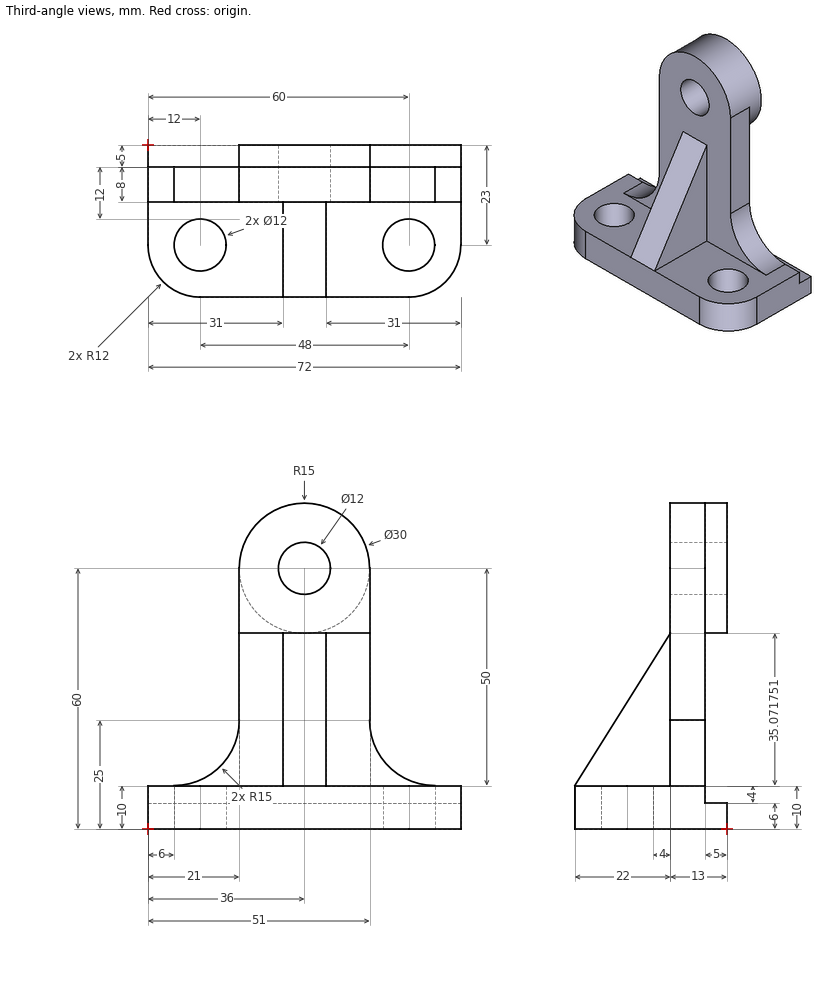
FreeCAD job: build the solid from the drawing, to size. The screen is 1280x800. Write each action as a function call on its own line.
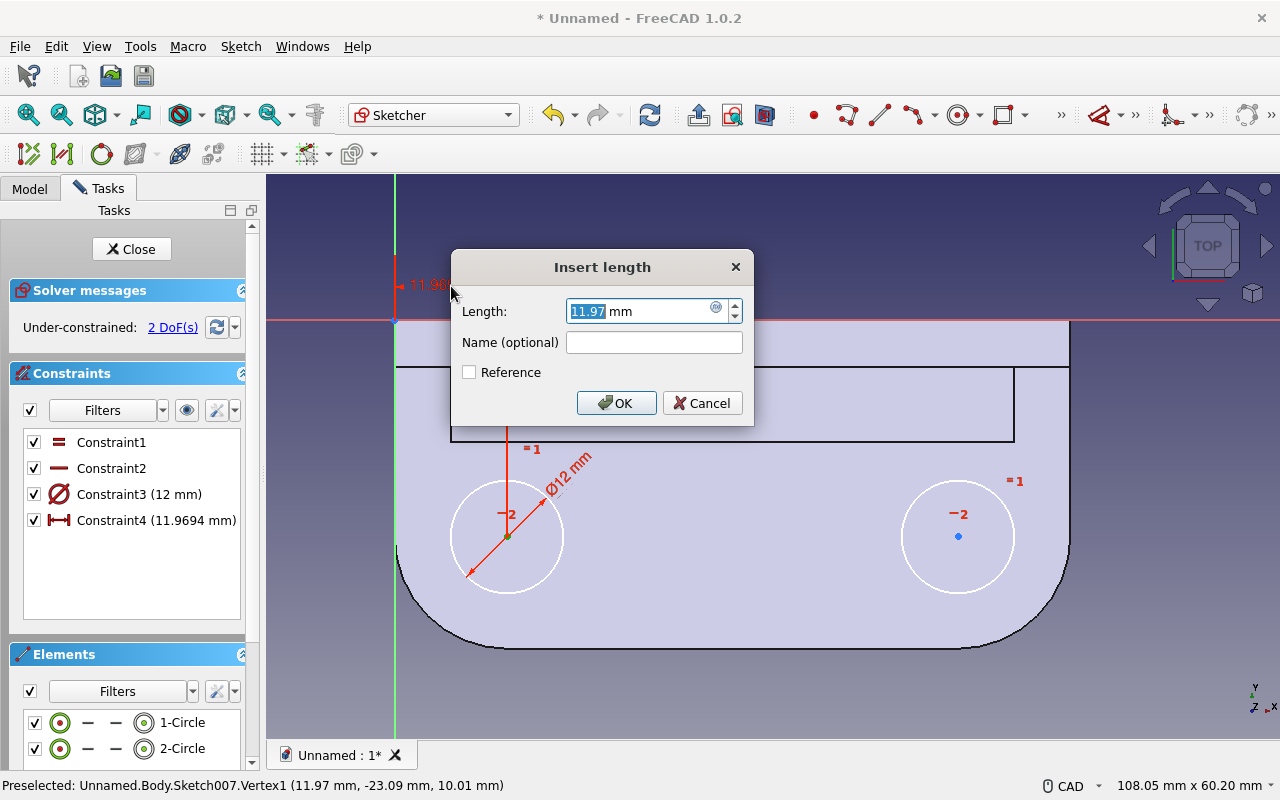
text(12)
key(Return)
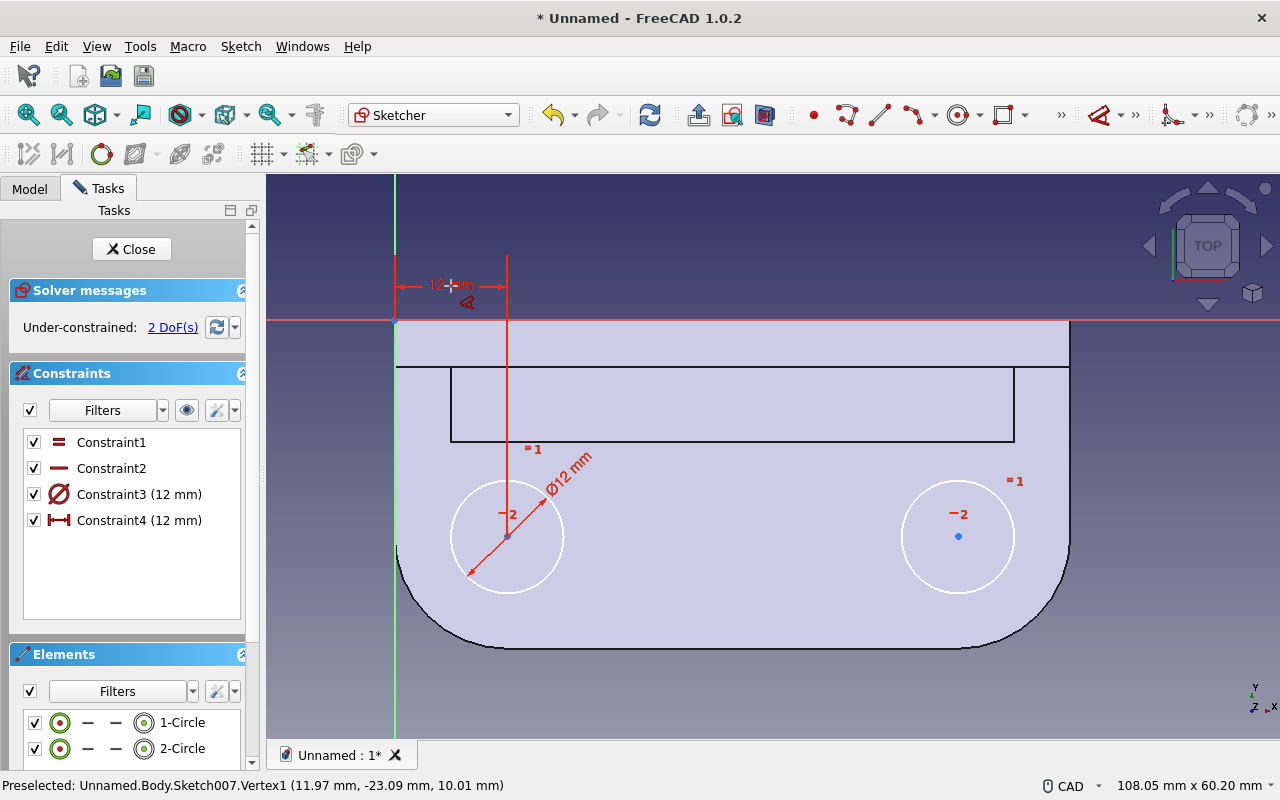
click(507, 537)
click(361, 429)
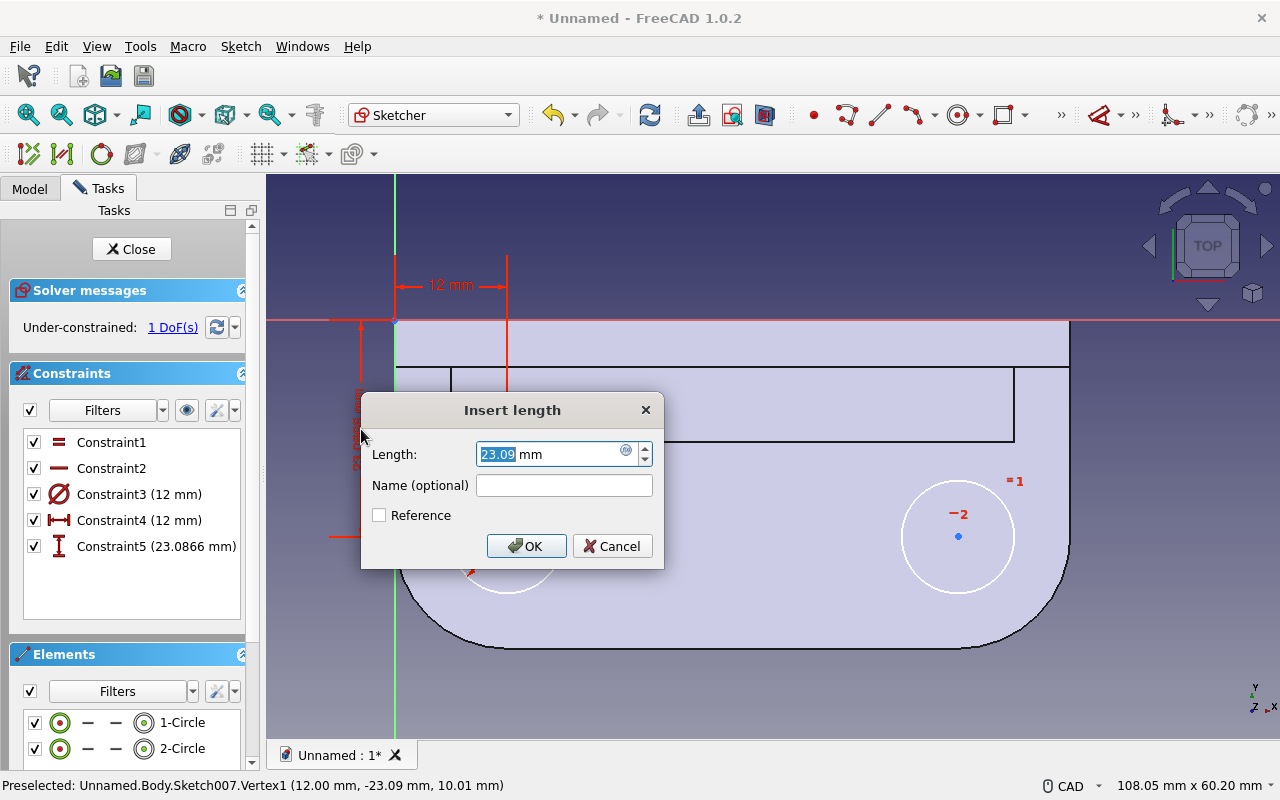
text(23)
key(Return)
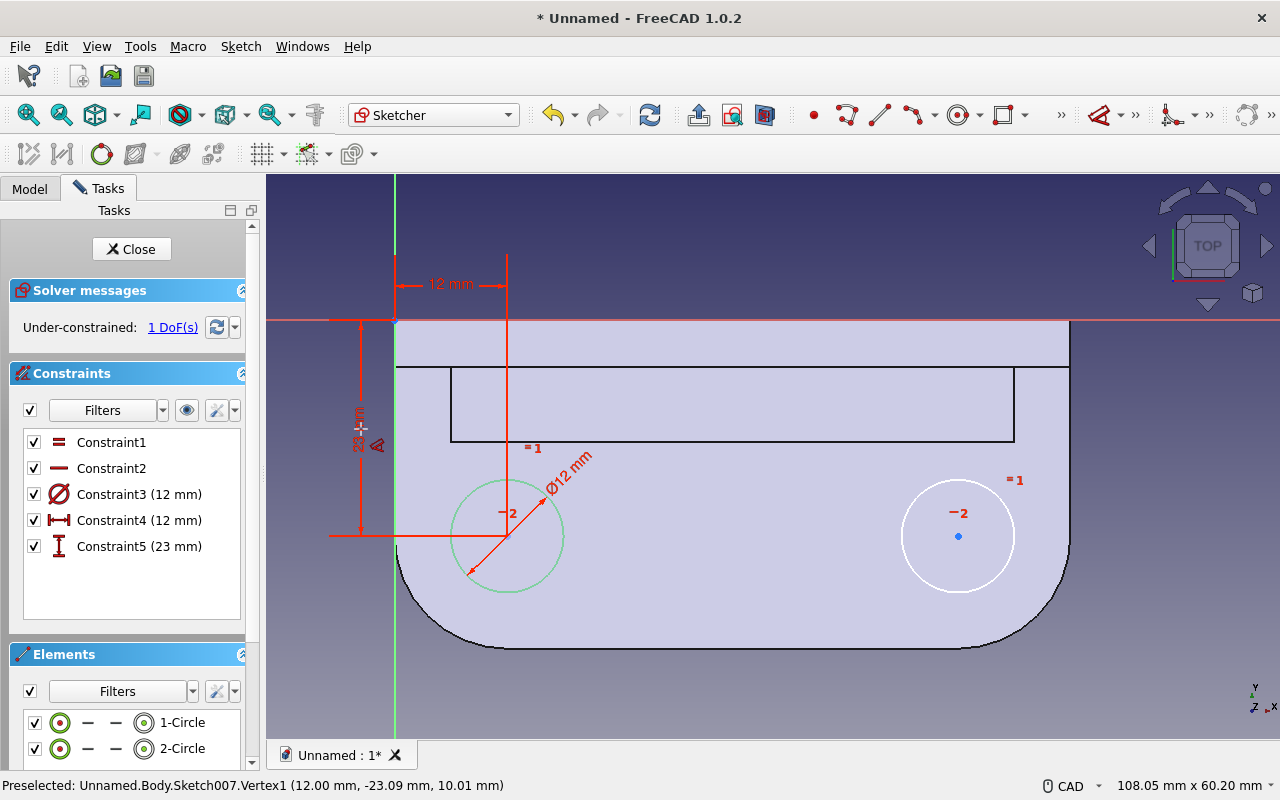
click(958, 536)
click(676, 286)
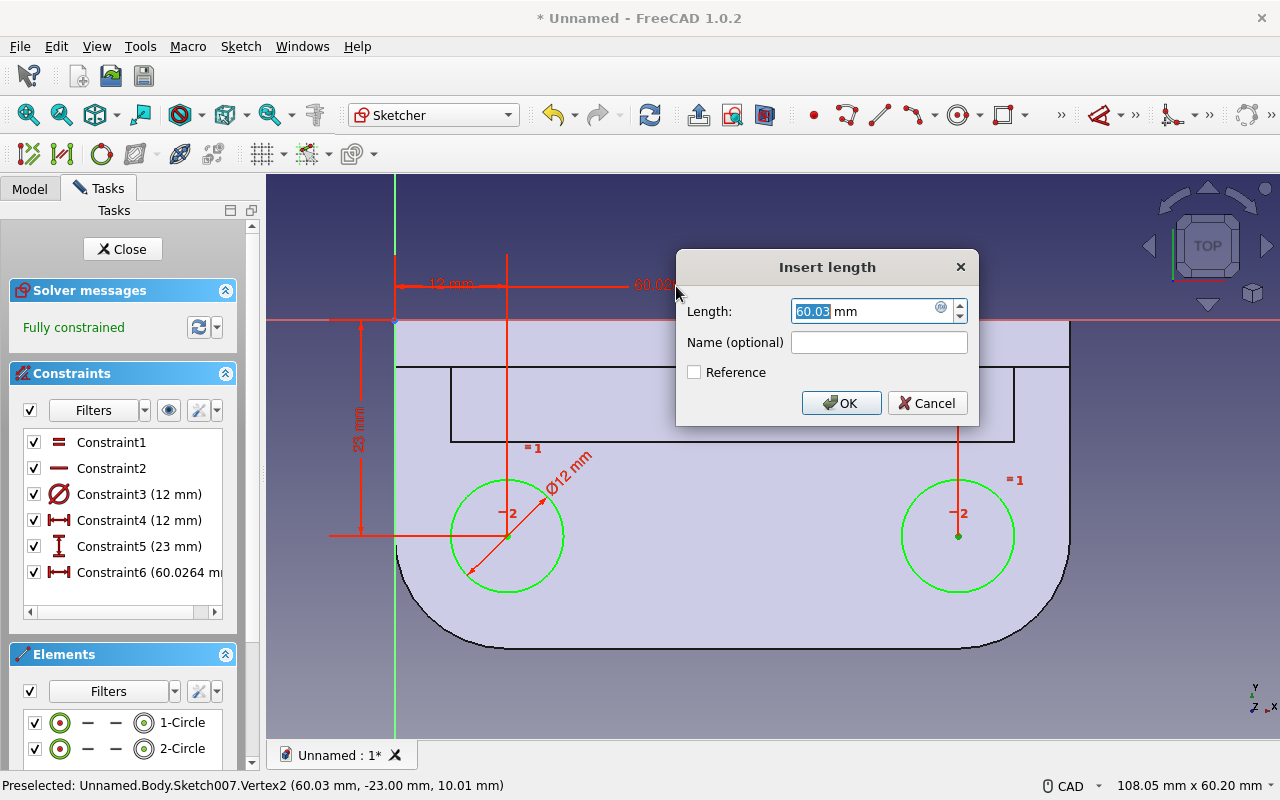
text(60)
key(Return)
key(Escape)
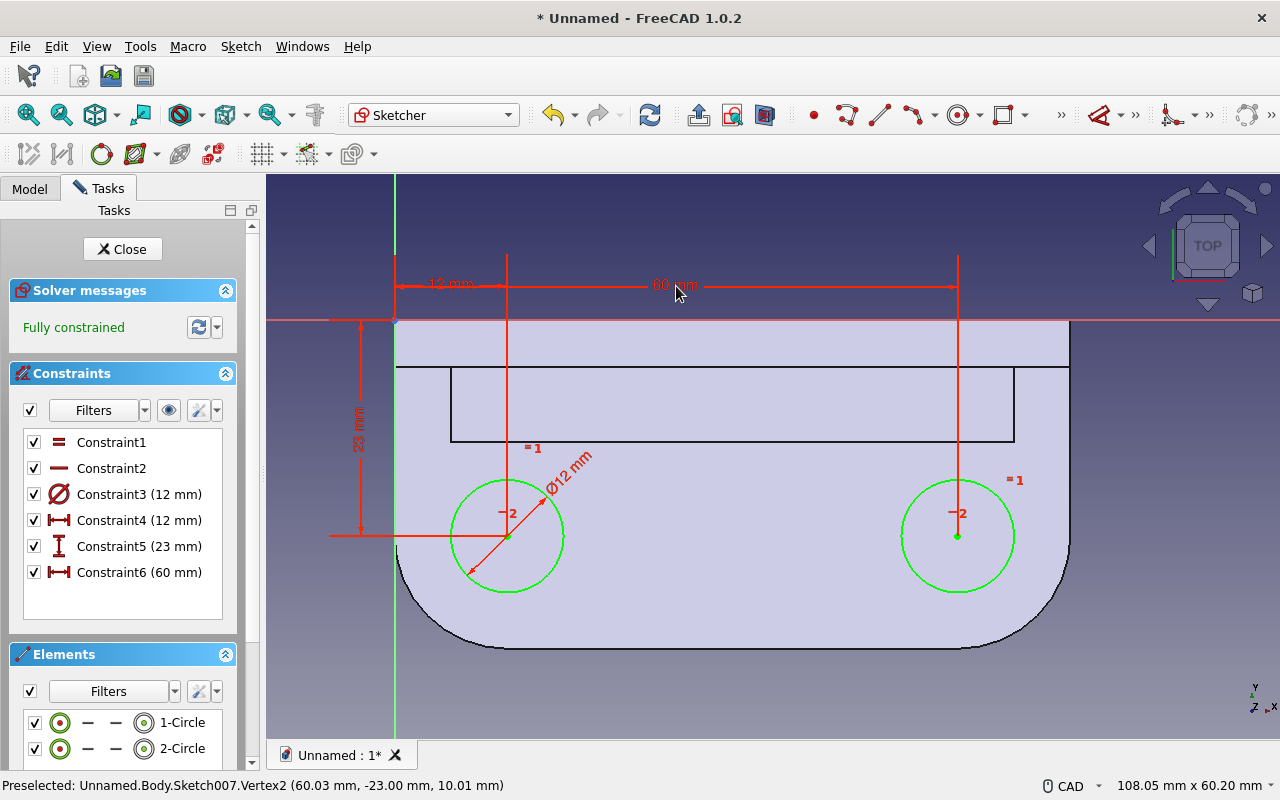
click(123, 249)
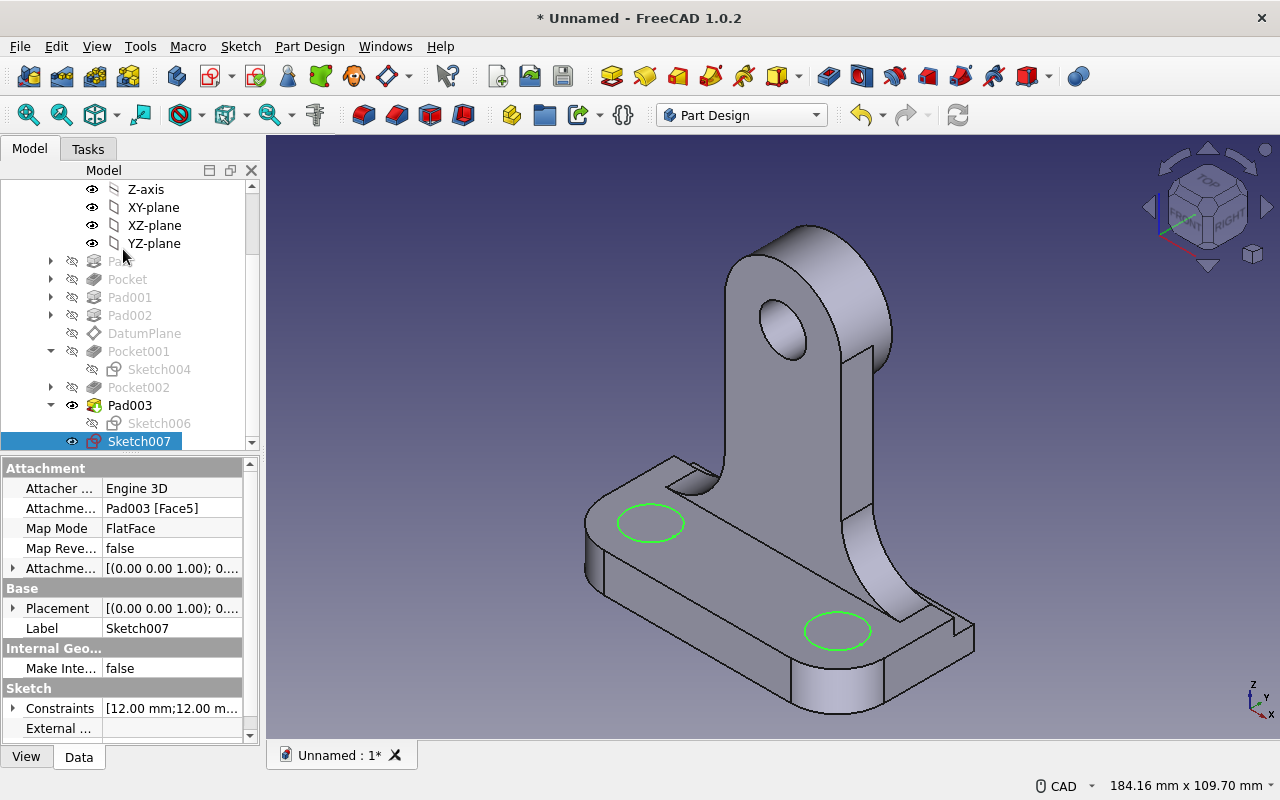
click(829, 76)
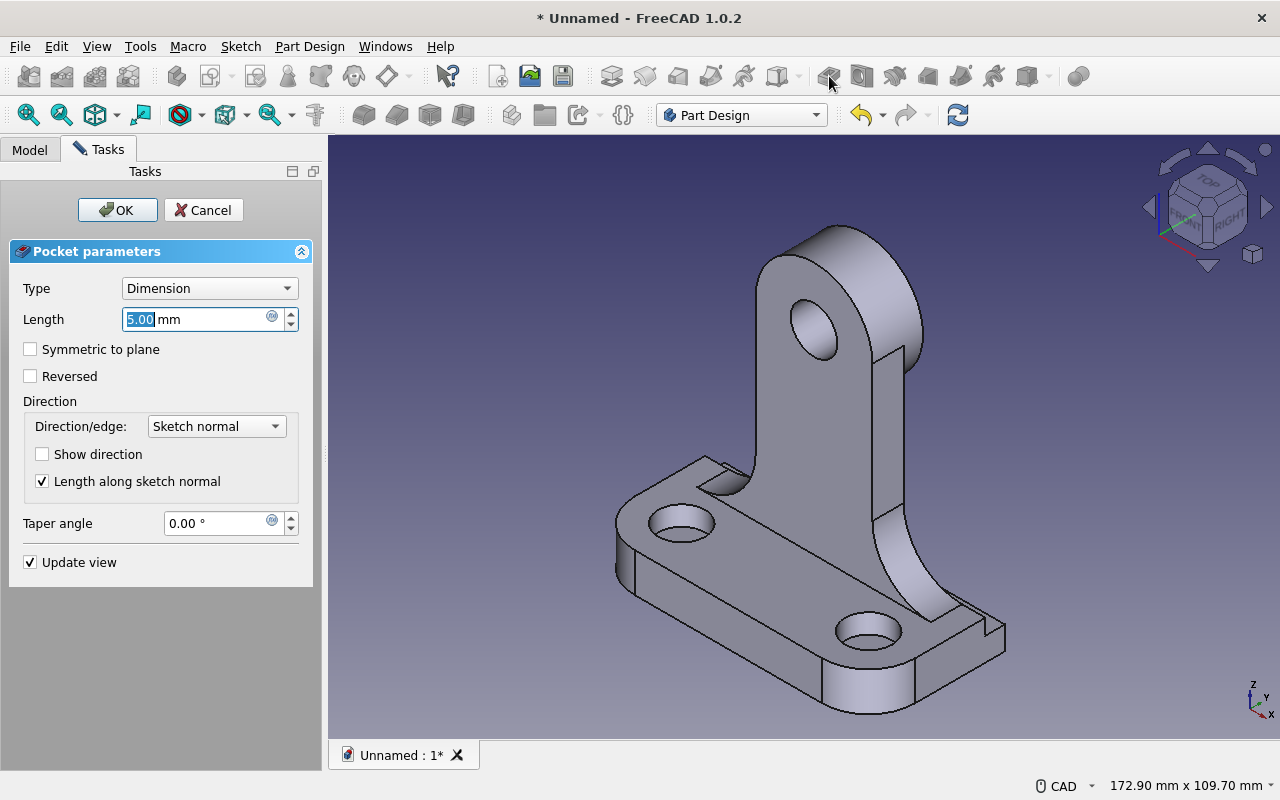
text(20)
key(Tab)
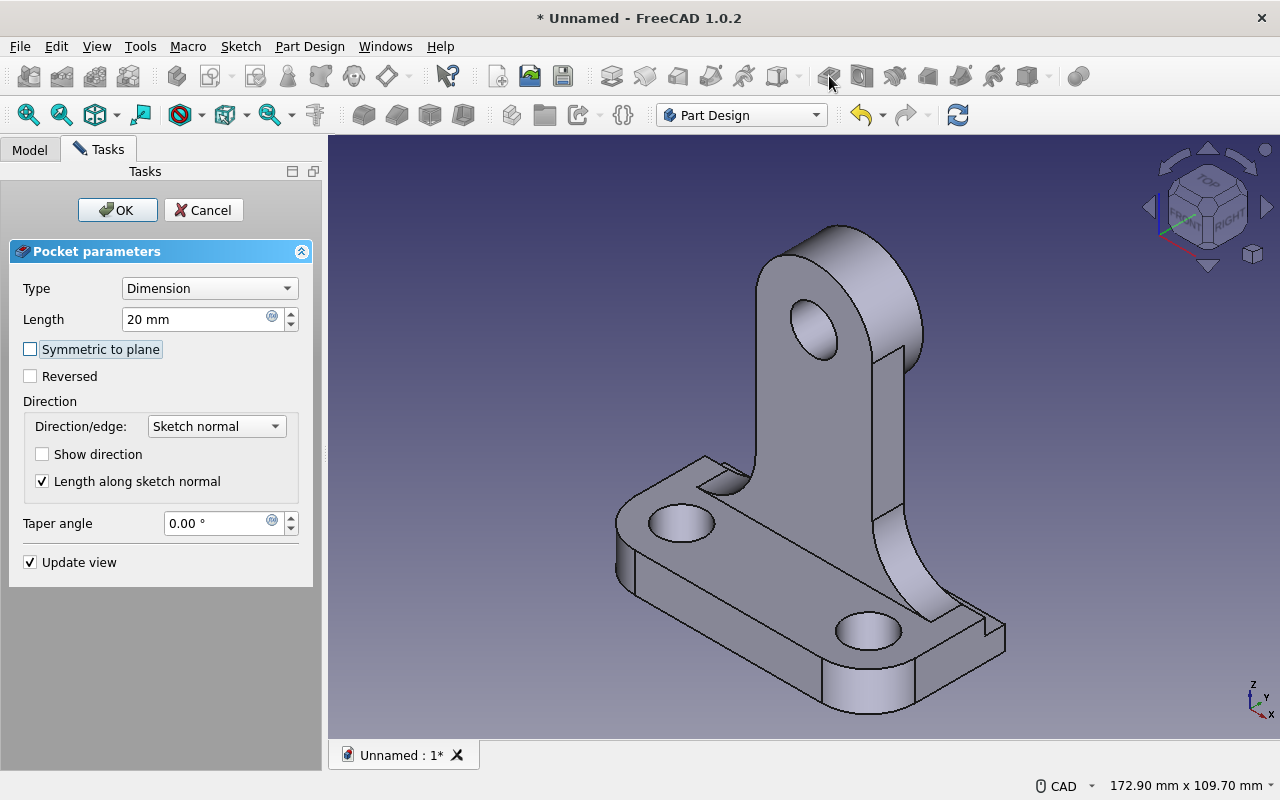
click(118, 210)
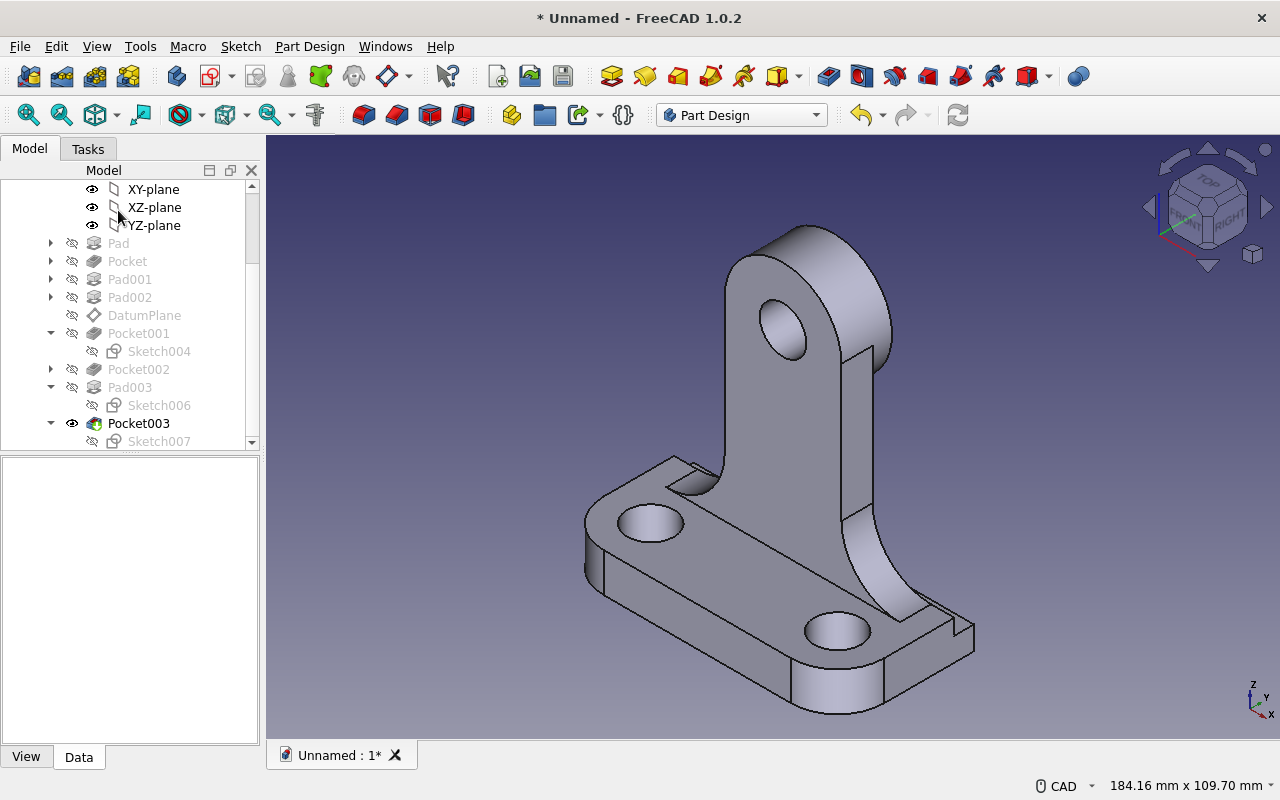
click(210, 76)